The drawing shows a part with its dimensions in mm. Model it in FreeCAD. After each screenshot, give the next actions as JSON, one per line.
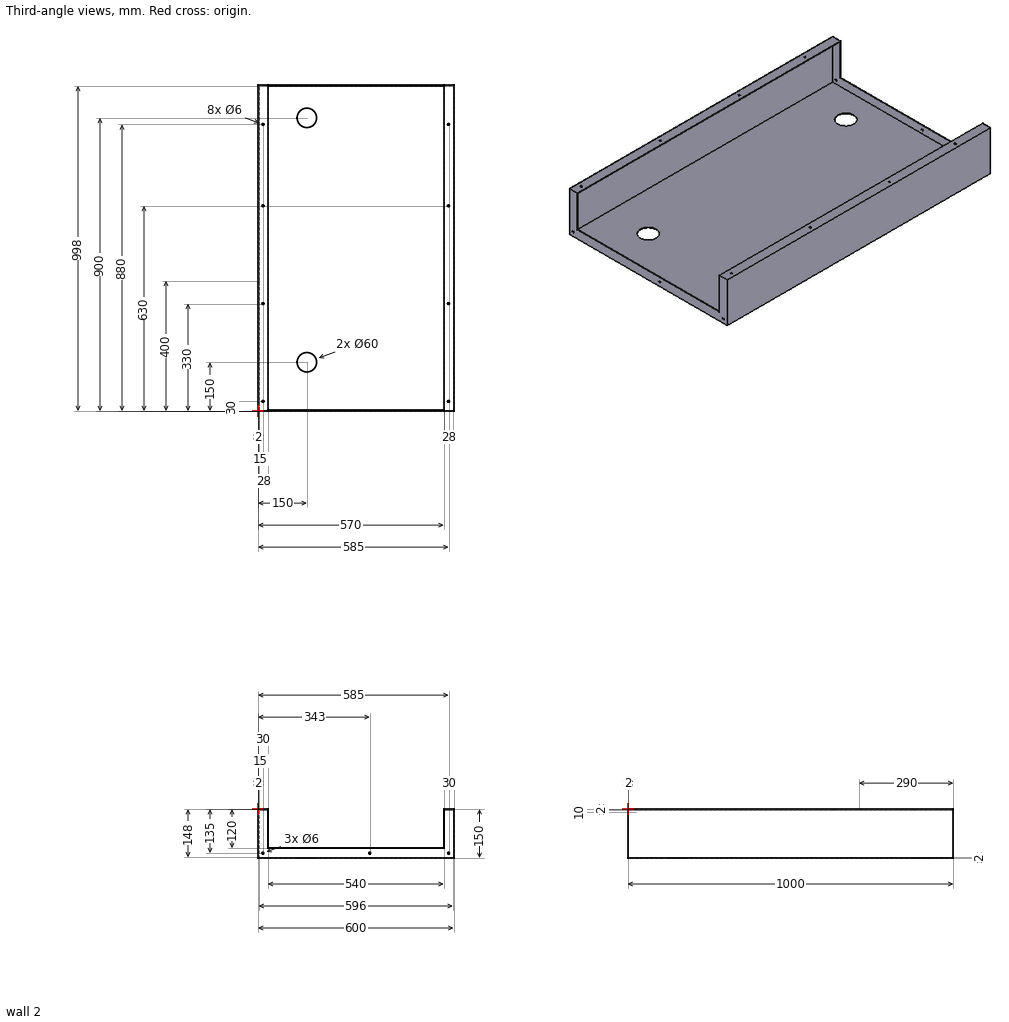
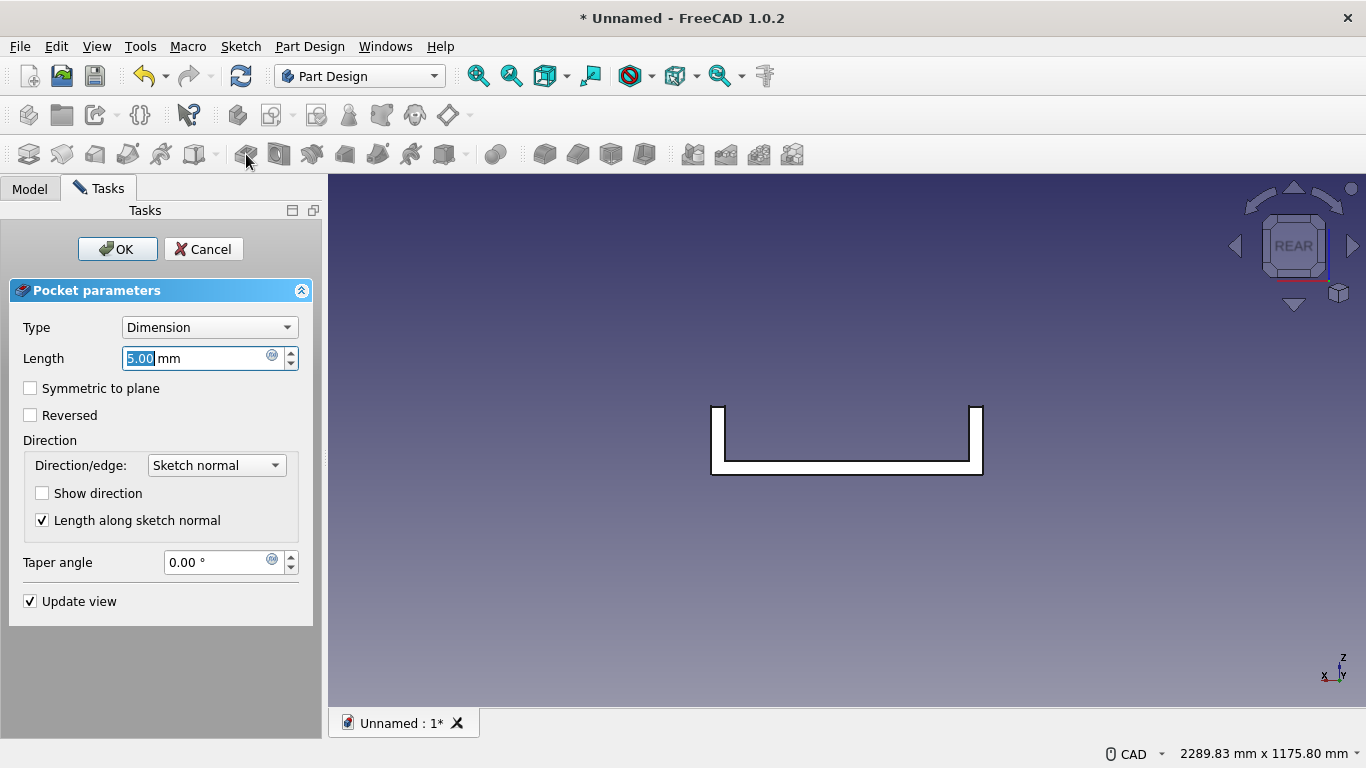
{"action": "type", "text": "290"}
{"action": "key", "text": "Tab"}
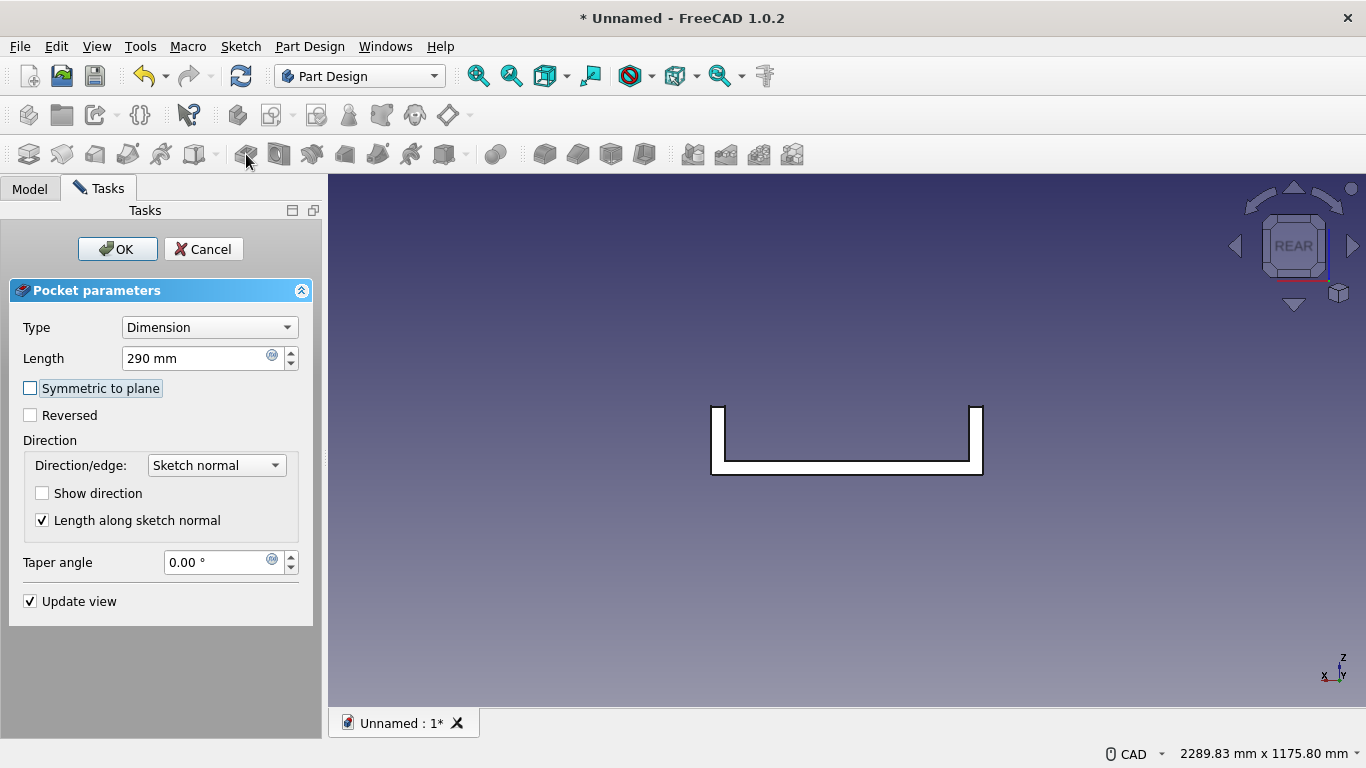
{"action": "left_click", "coordinate": [118, 249]}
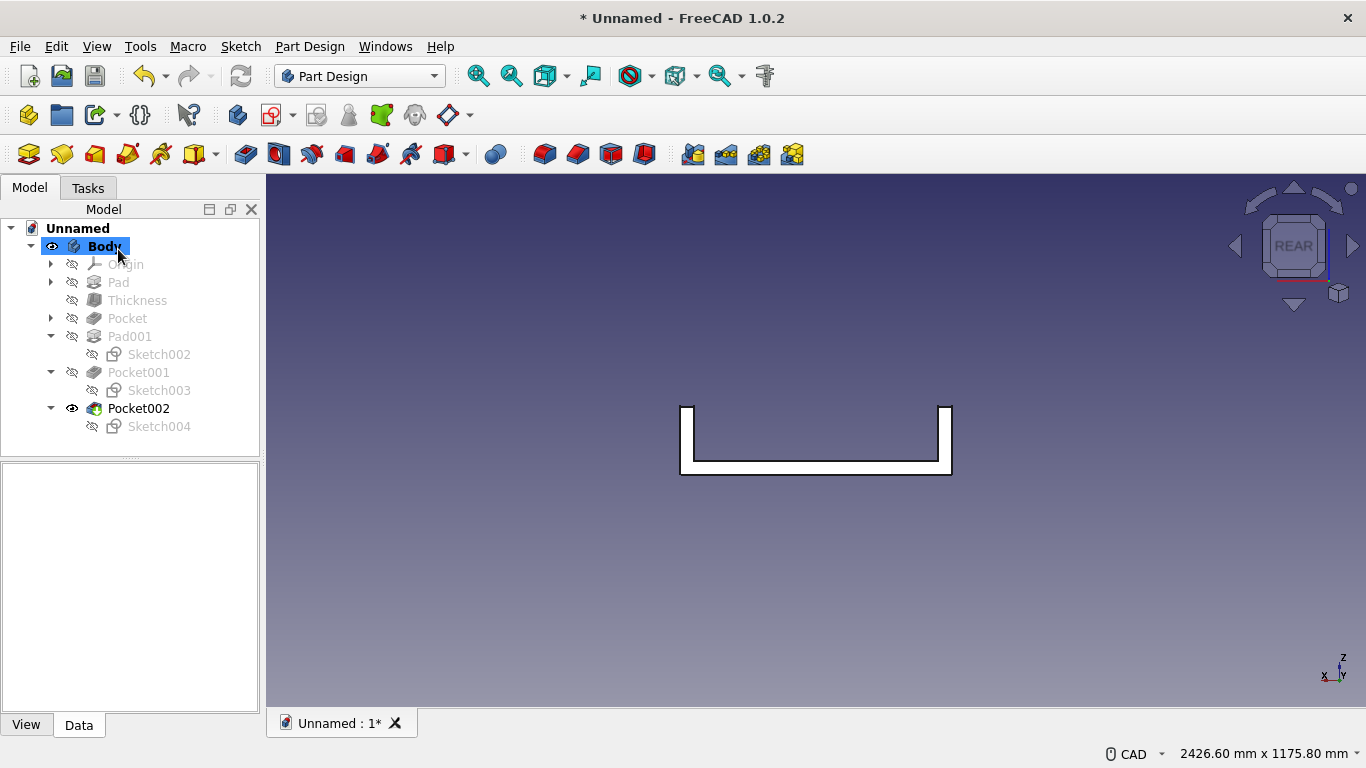
{"action": "left_click", "coordinate": [479, 76]}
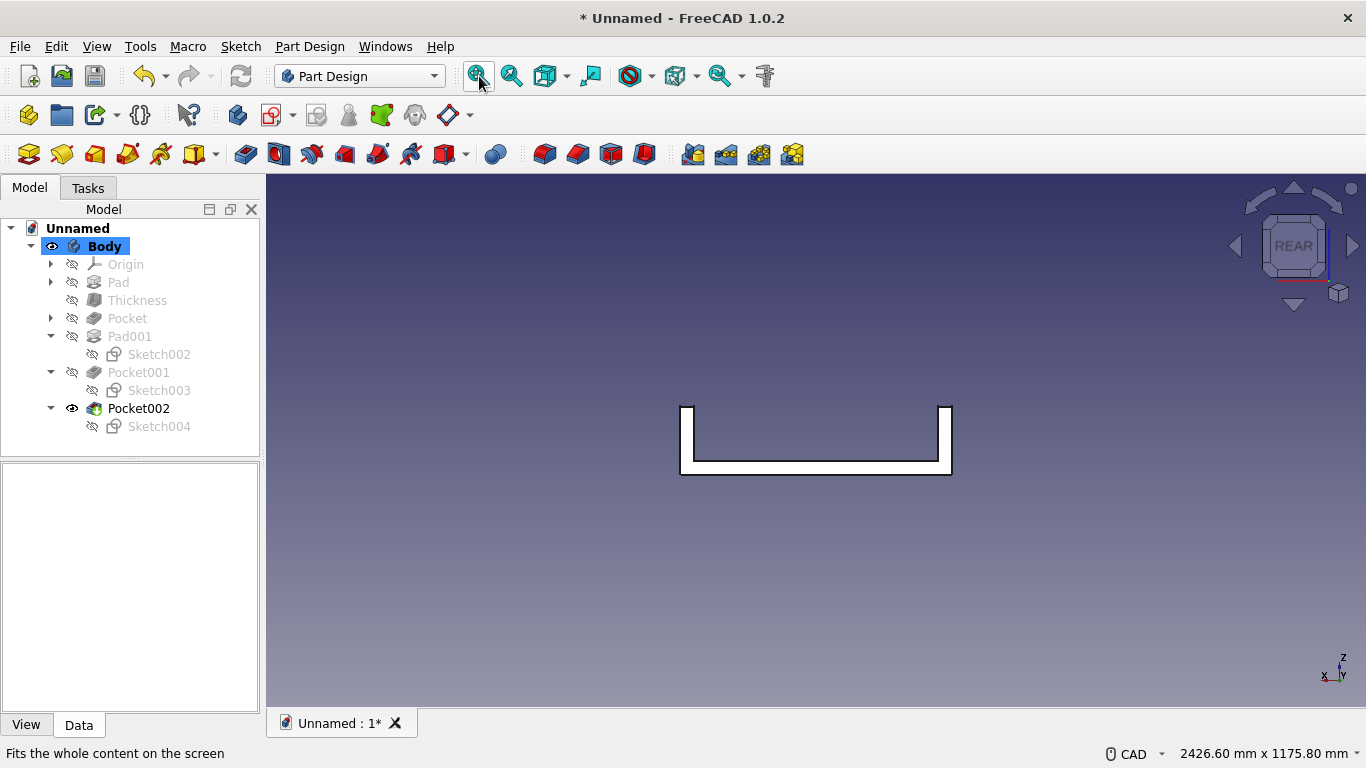
{"action": "left_click", "coordinate": [270, 116]}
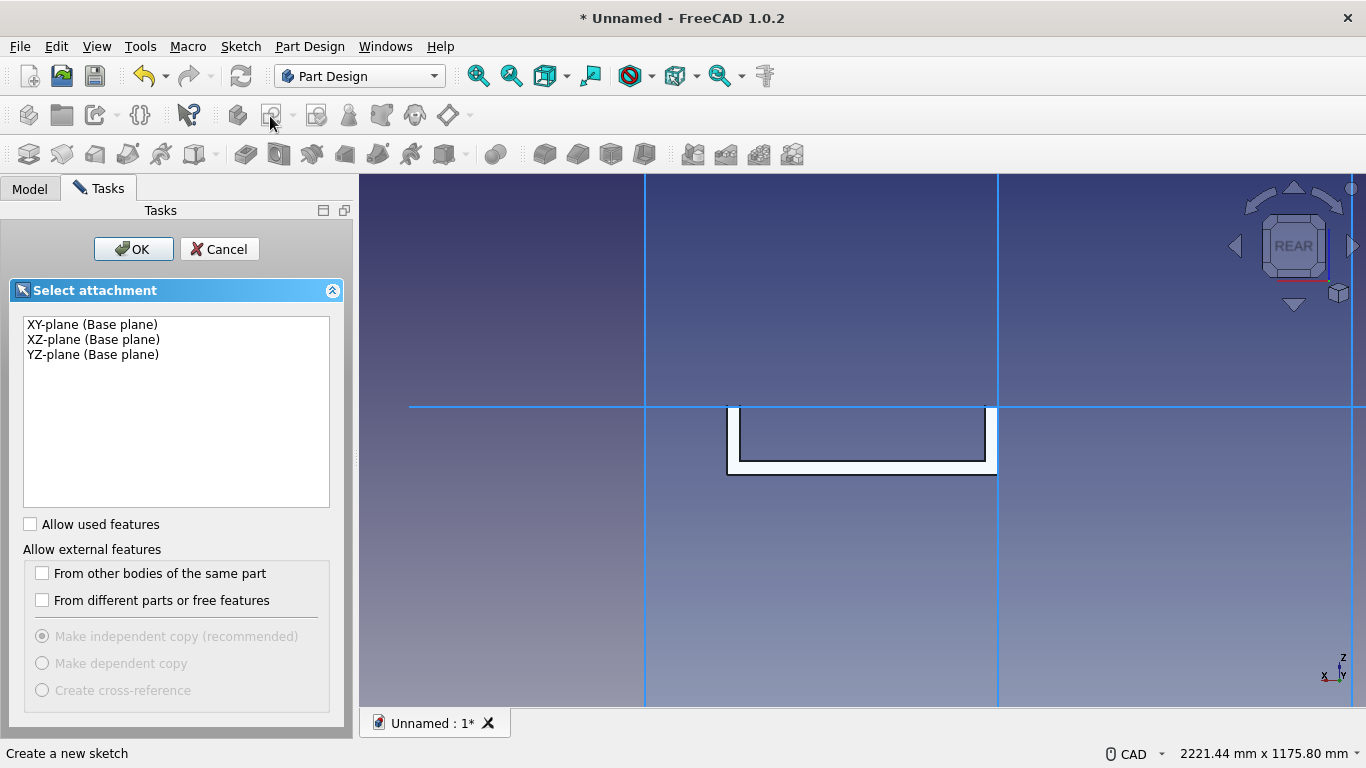
{"action": "left_click", "coordinate": [84, 340]}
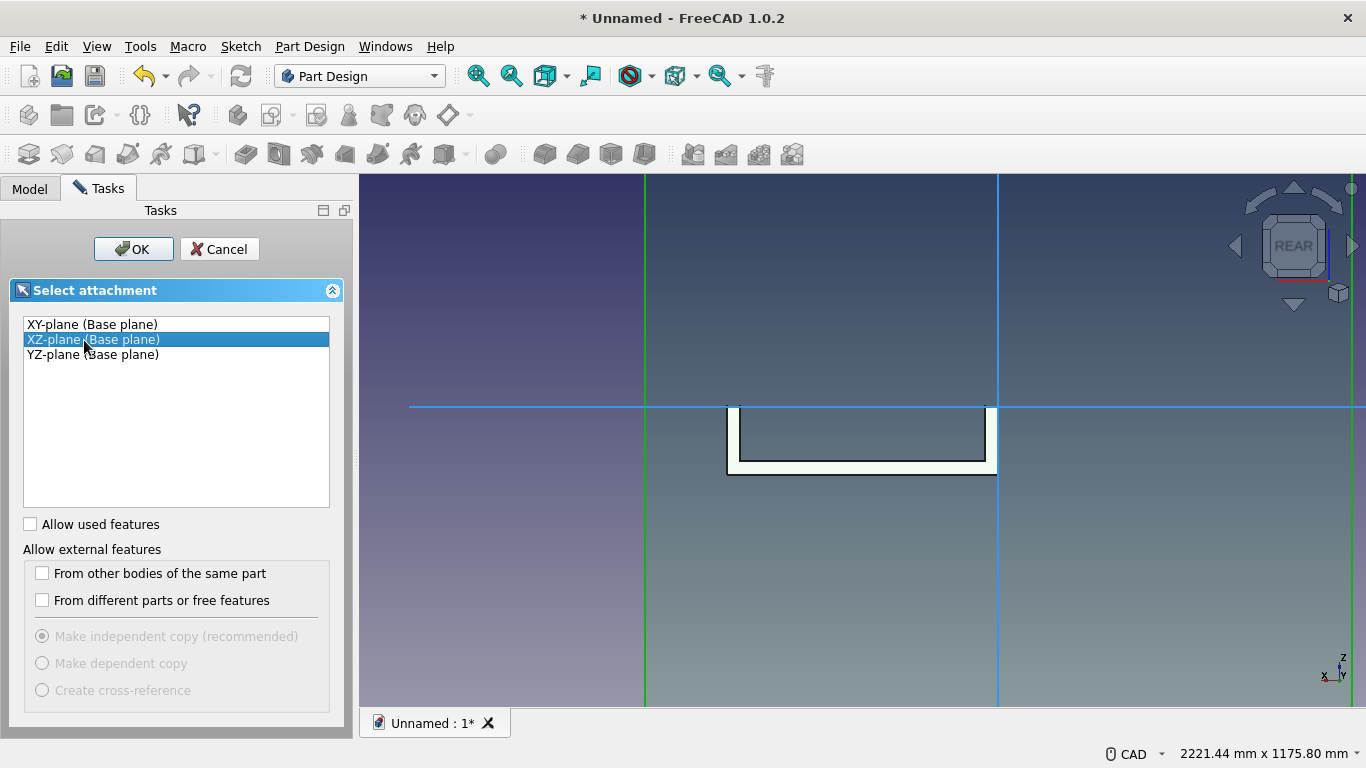
{"action": "left_click", "coordinate": [134, 249]}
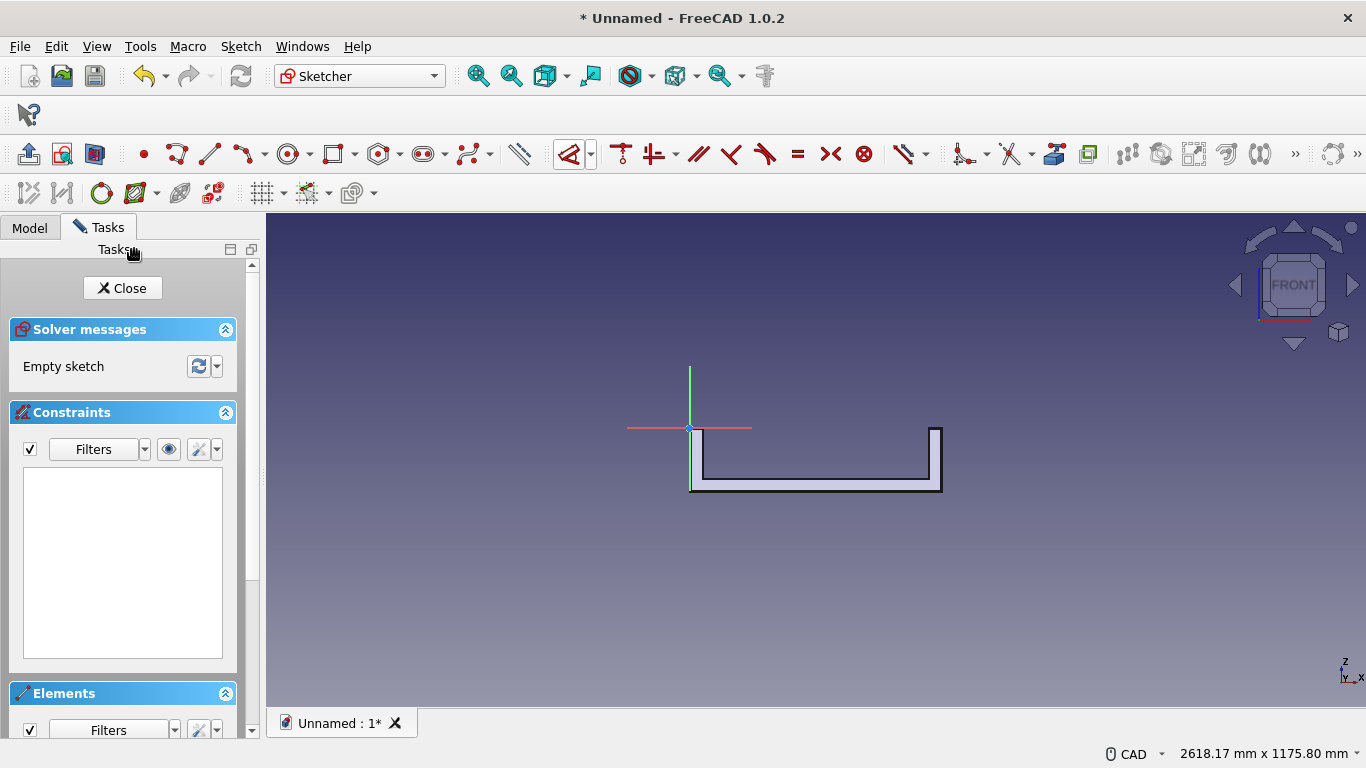
{"action": "scroll", "coordinate": [856, 460], "scroll_direction": "up", "scroll_amount": 5}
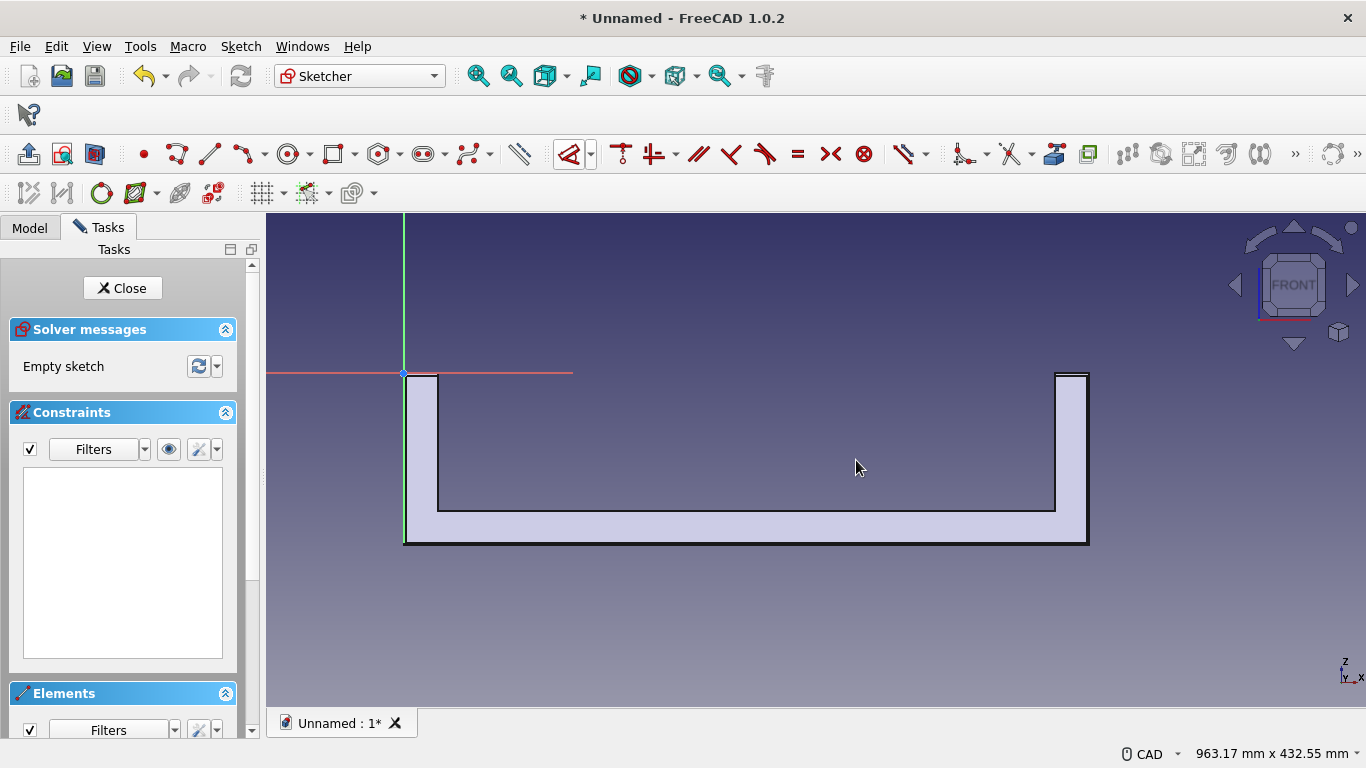
{"action": "left_click", "coordinate": [177, 154]}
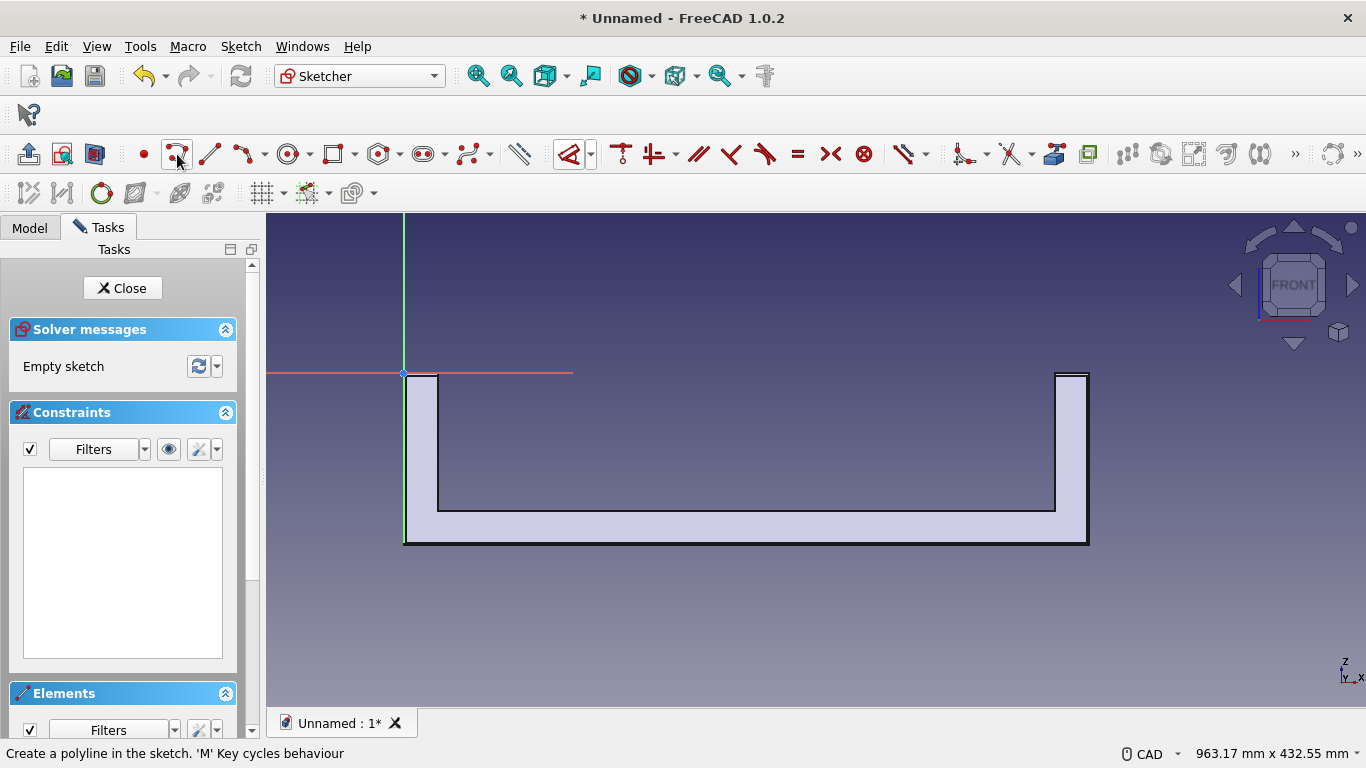
{"action": "left_click", "coordinate": [404, 373]}
{"action": "left_click", "coordinate": [413, 545]}
{"action": "left_click", "coordinate": [1089, 545]}
{"action": "left_click", "coordinate": [1089, 373]}
{"action": "left_click", "coordinate": [1055, 382]}
{"action": "left_click", "coordinate": [1055, 511]}
{"action": "left_click", "coordinate": [438, 511]}
{"action": "left_click", "coordinate": [438, 382]}
{"action": "left_click", "coordinate": [404, 373]}
{"action": "key", "text": "Escape"}
{"action": "key", "text": "Escape"}